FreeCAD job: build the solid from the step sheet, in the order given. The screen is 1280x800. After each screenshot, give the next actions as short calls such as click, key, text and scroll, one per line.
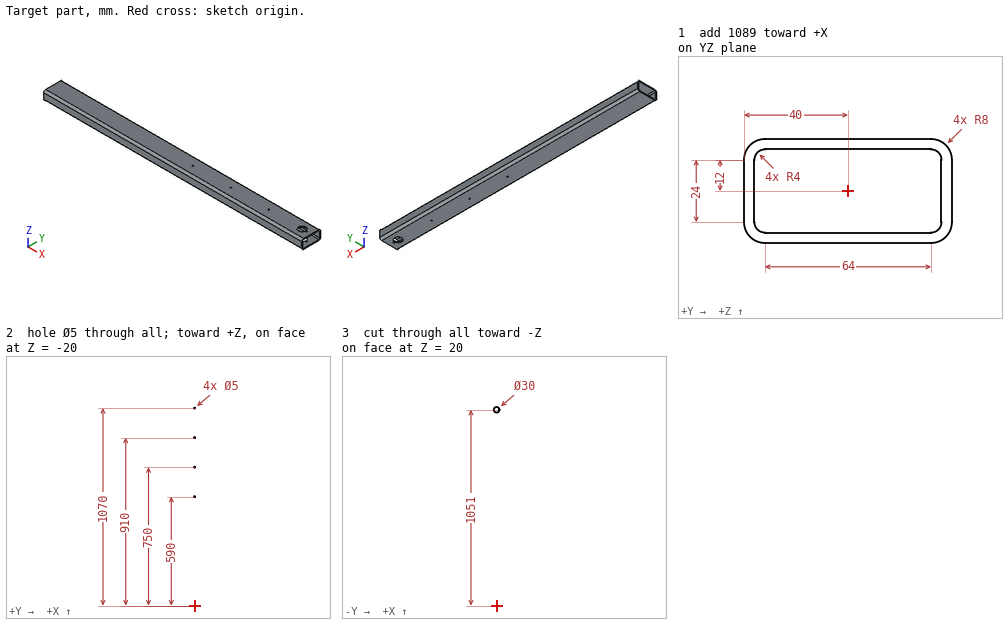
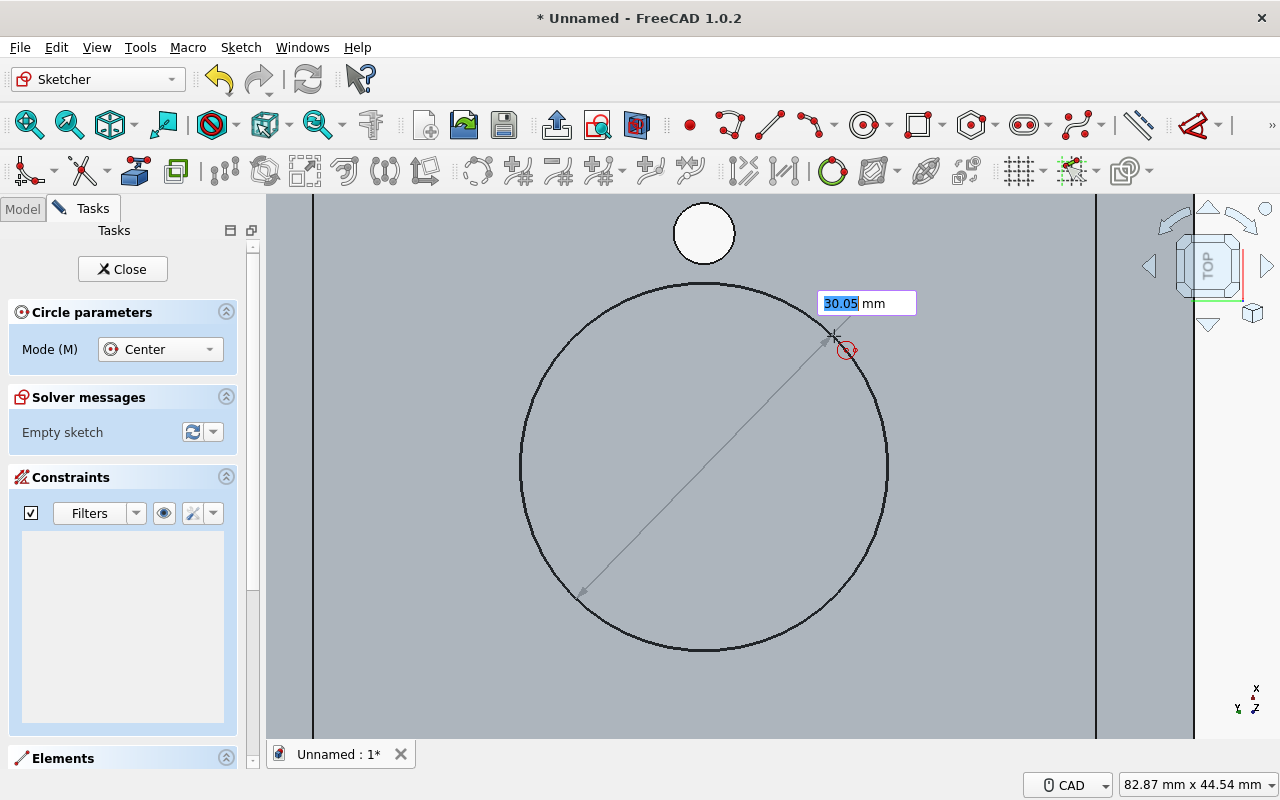
text(30)
key(Return)
key(Escape)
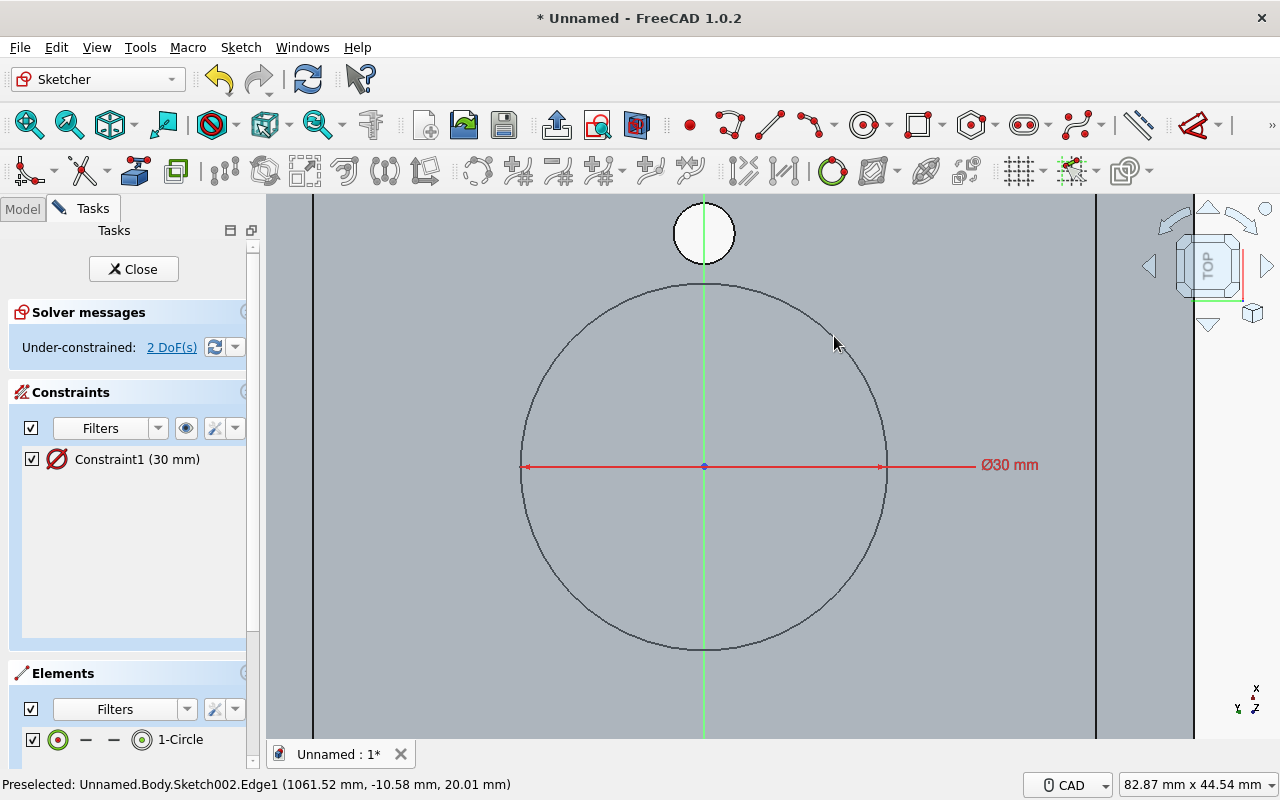
click(704, 467)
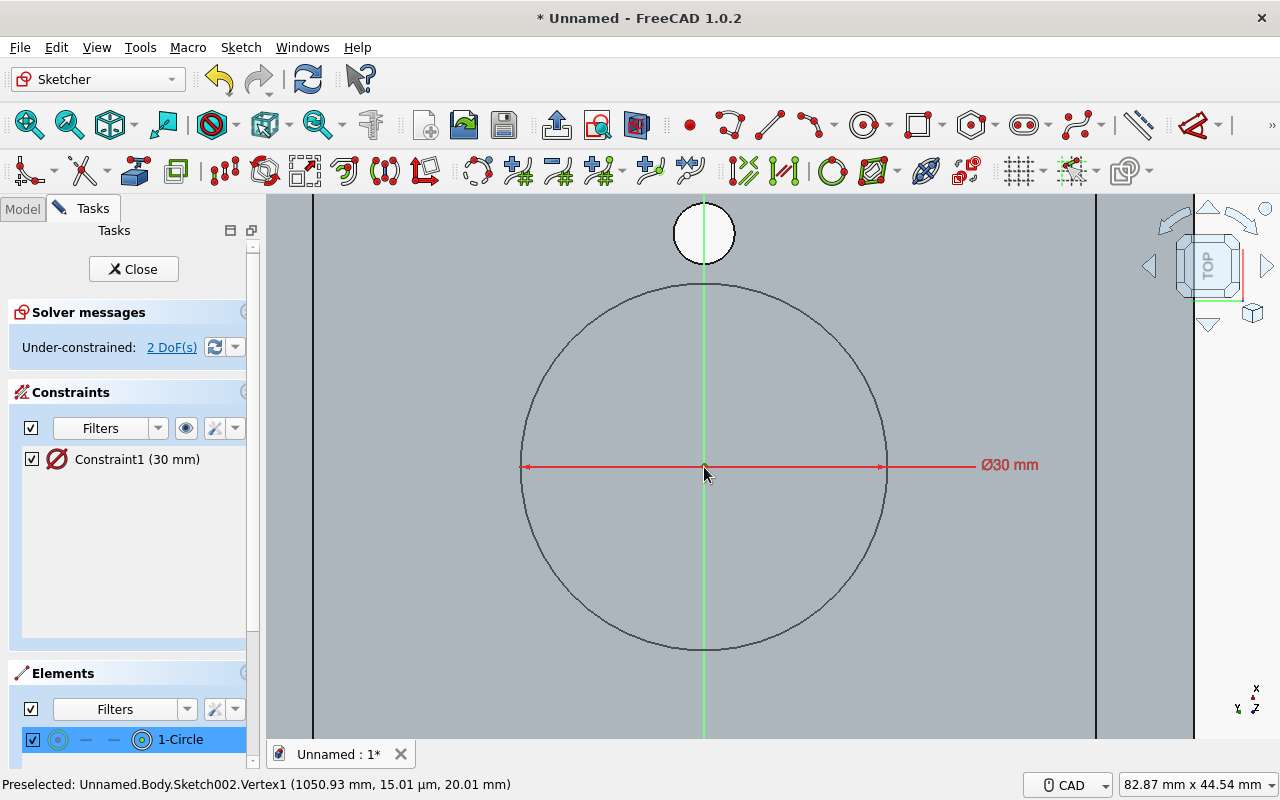
click(704, 606)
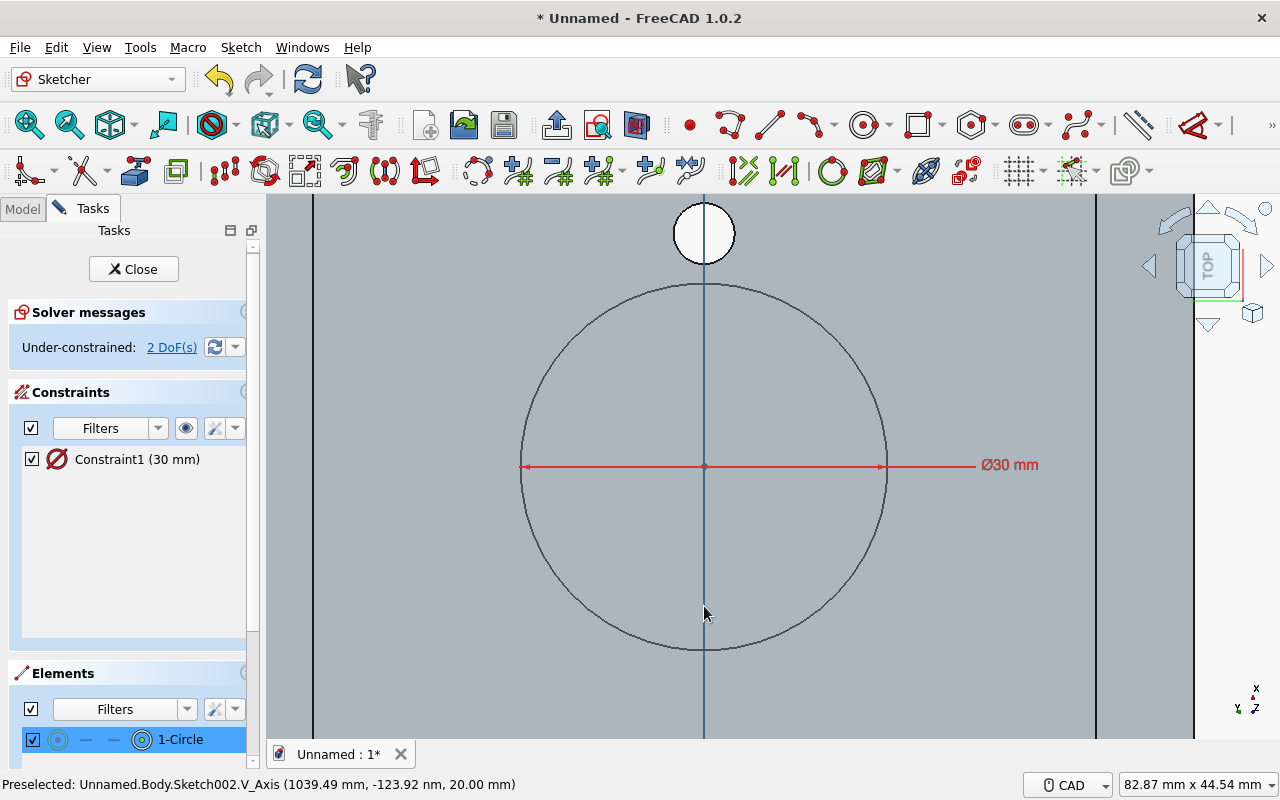
key(c)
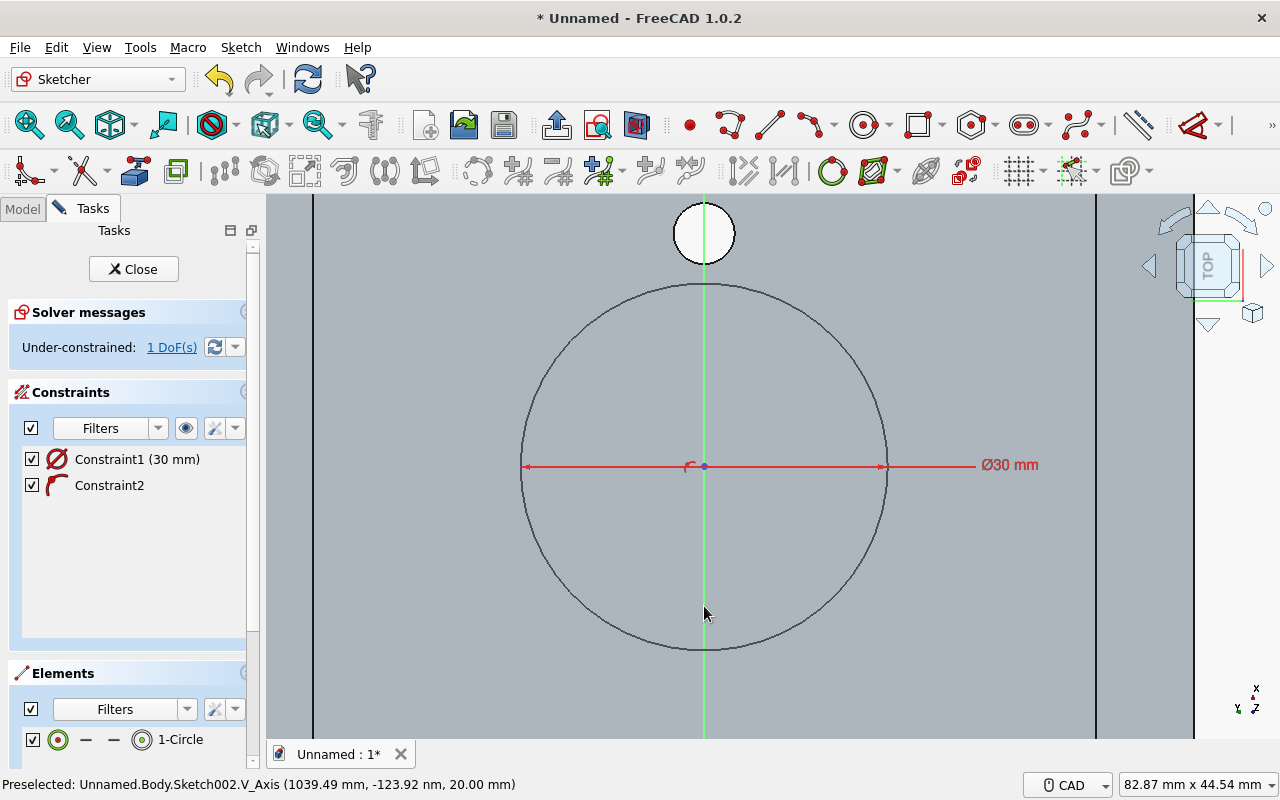
click(1194, 126)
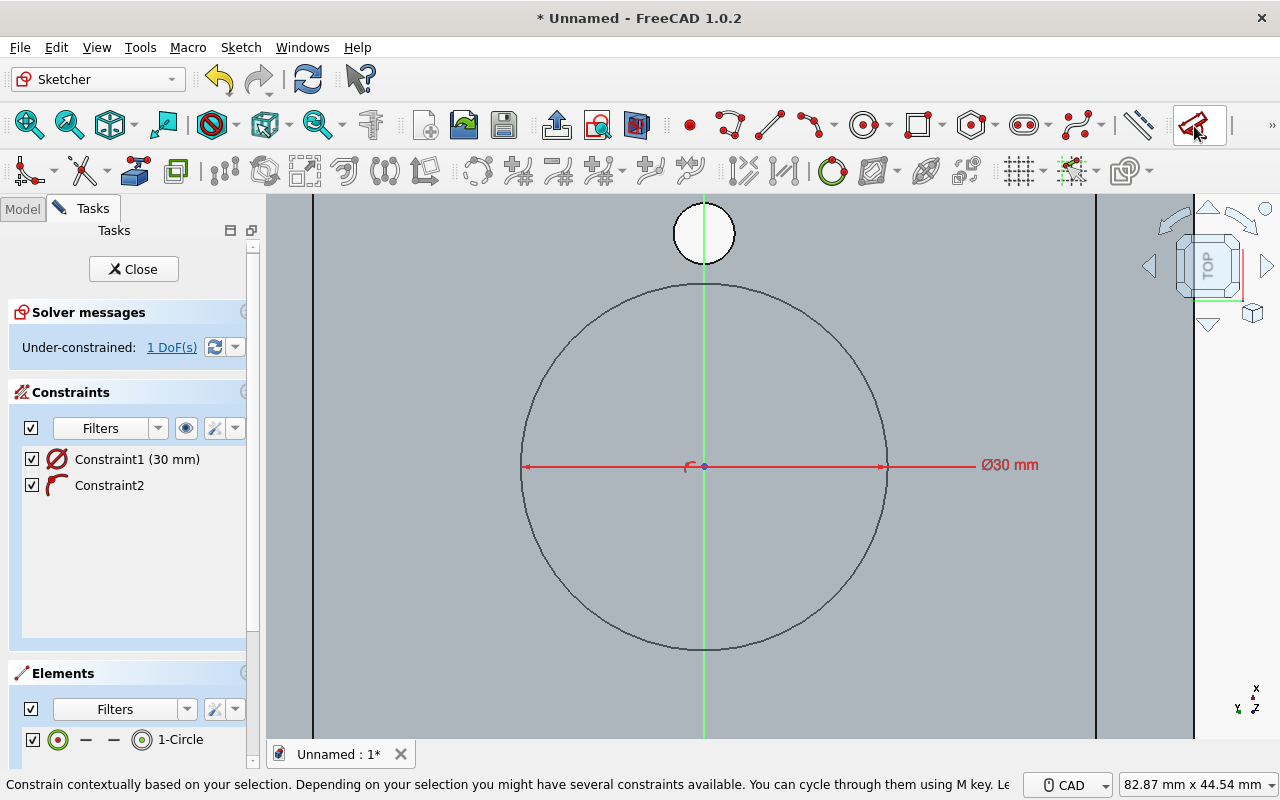
click(704, 467)
click(738, 589)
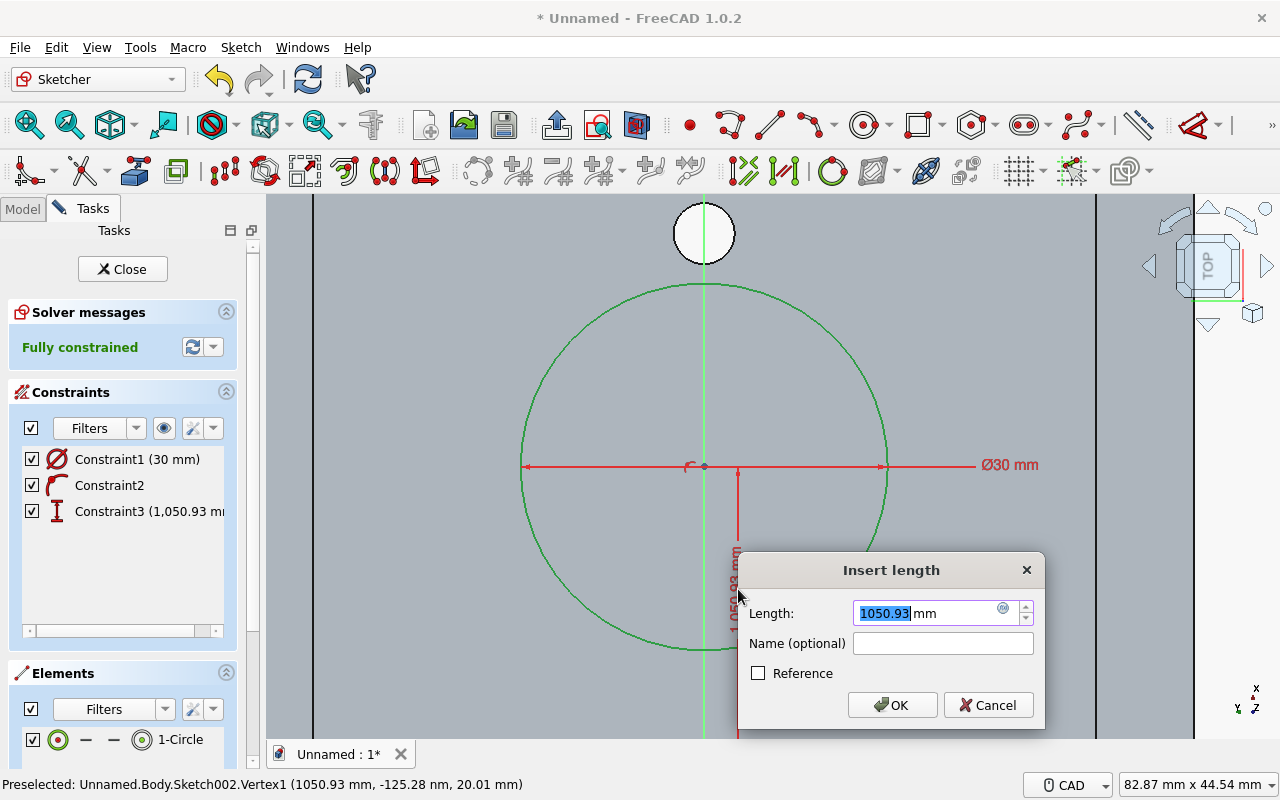
text(1051)
key(Return)
key(Escape)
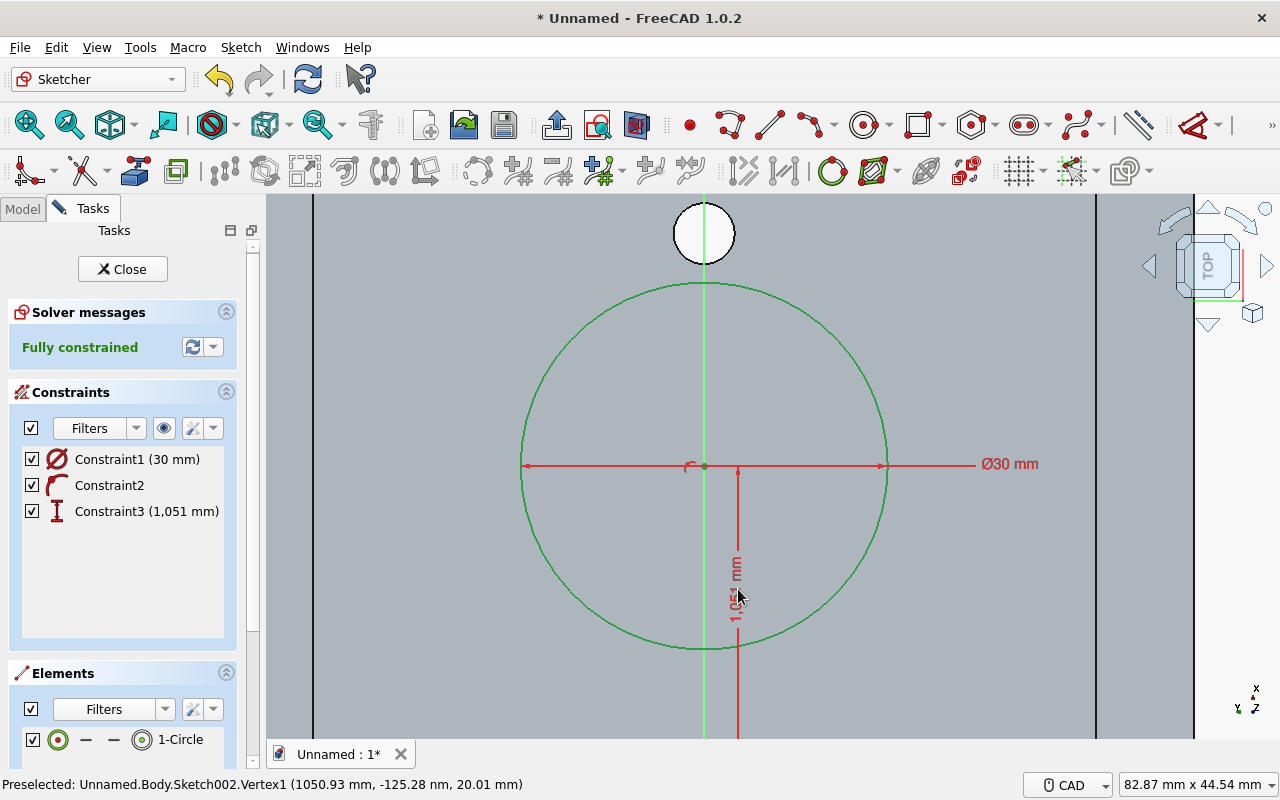
click(123, 269)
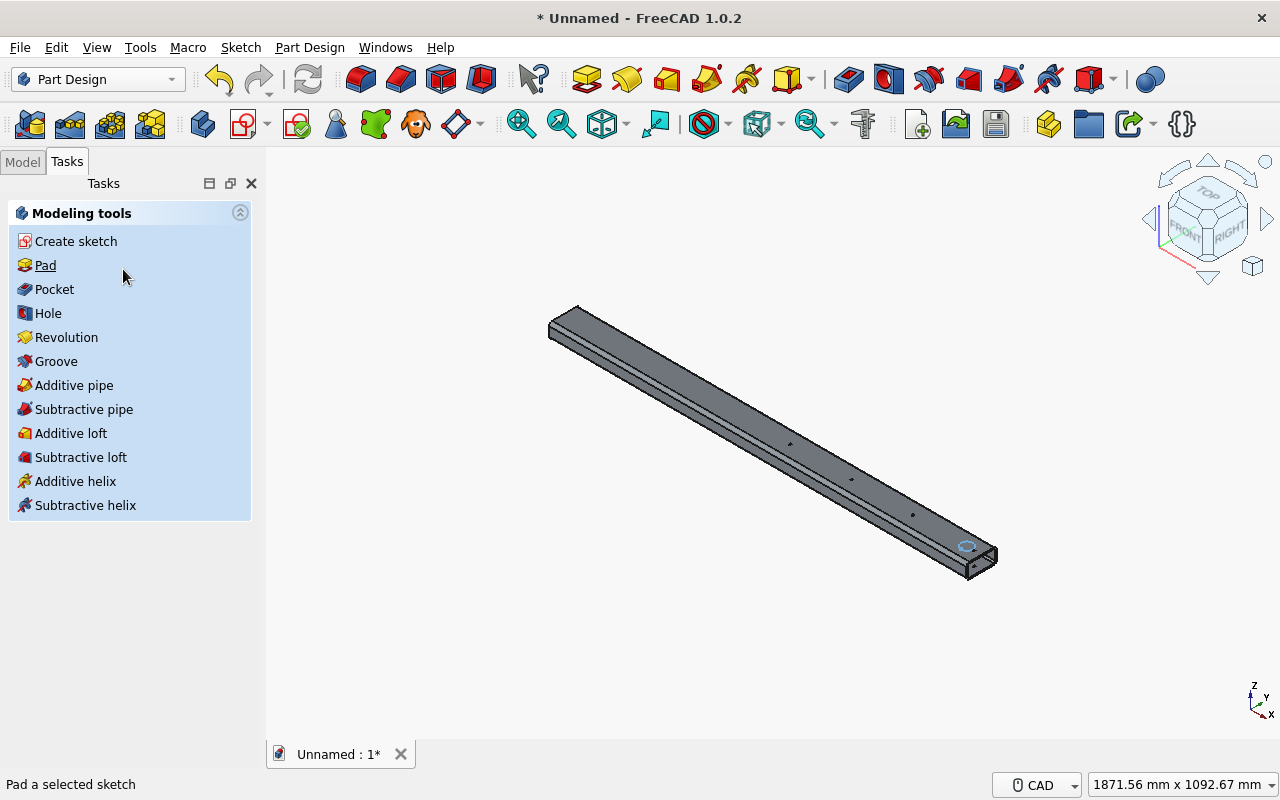
click(850, 80)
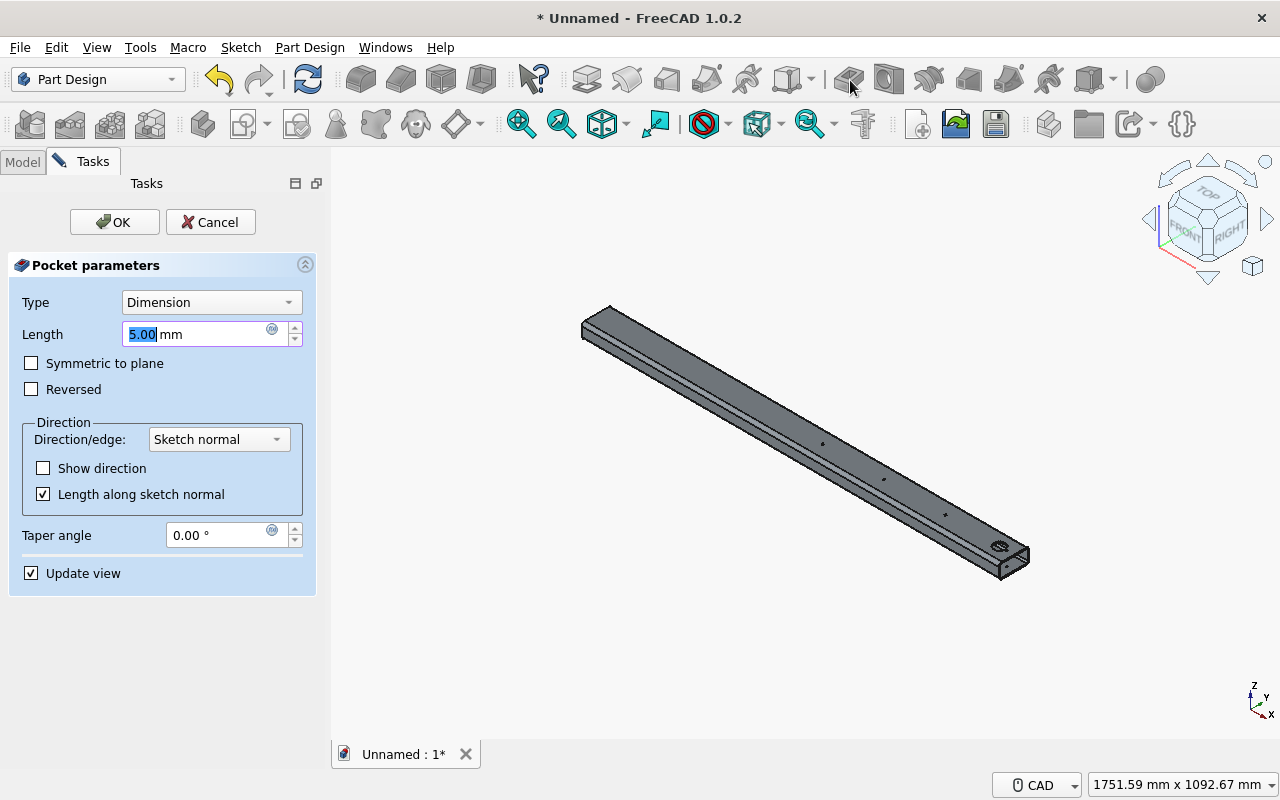
click(212, 302)